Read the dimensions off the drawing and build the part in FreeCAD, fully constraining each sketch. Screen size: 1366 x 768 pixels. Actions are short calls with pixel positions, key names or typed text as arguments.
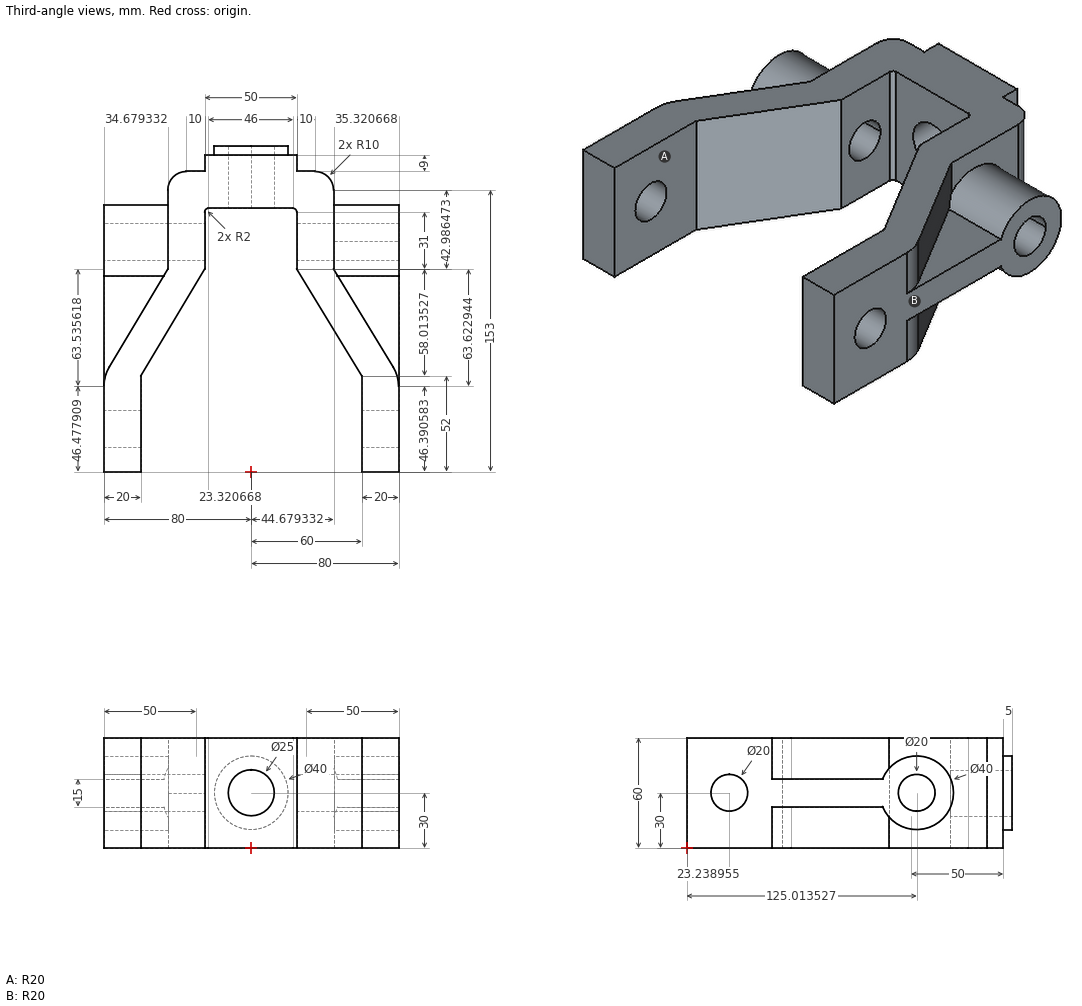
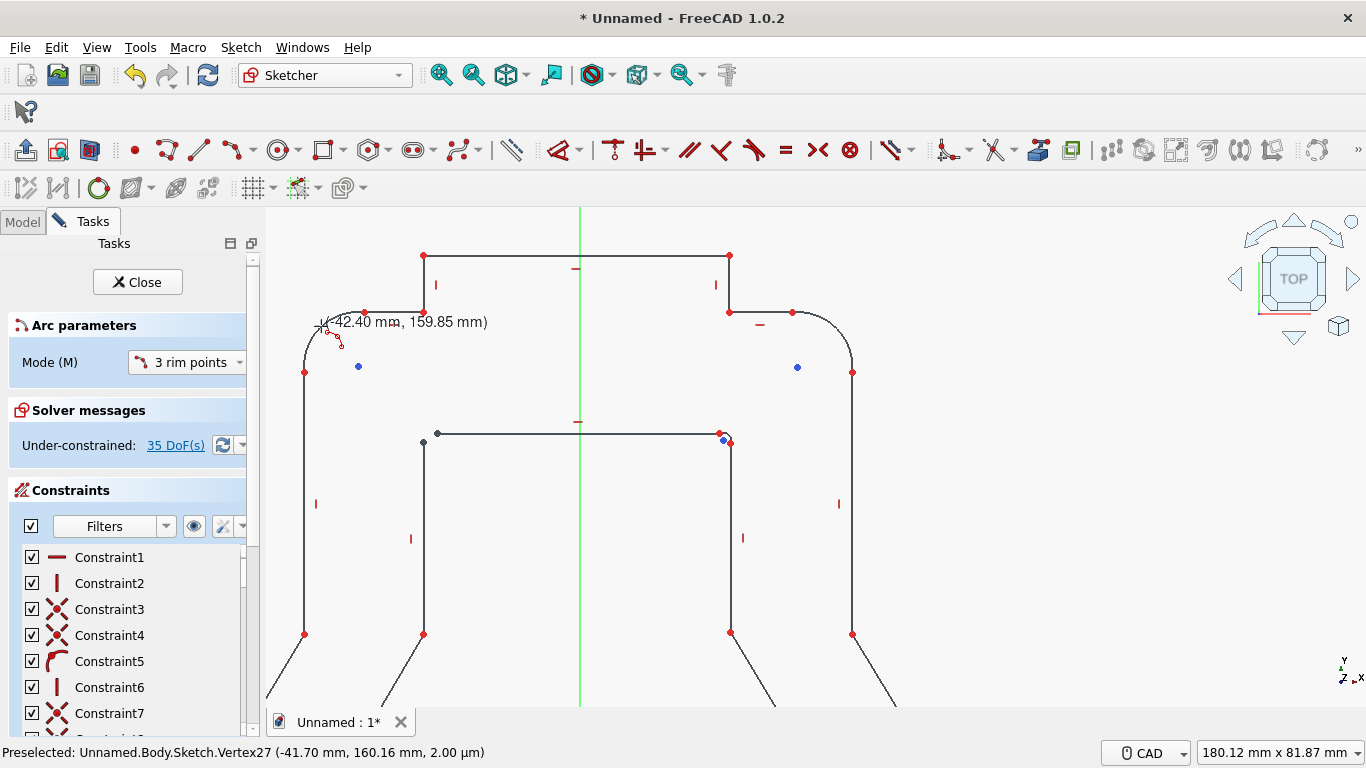
click(424, 443)
click(437, 434)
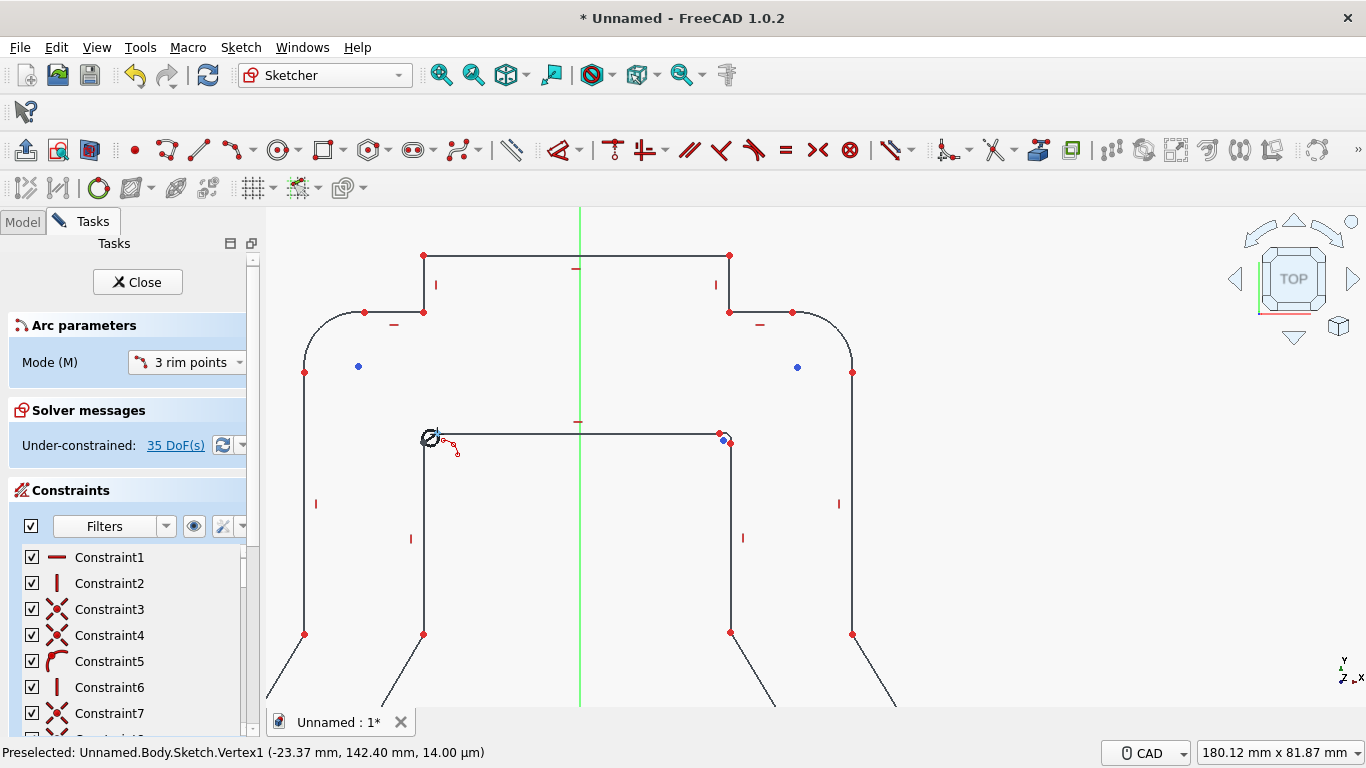
scroll(429, 433, up, 8)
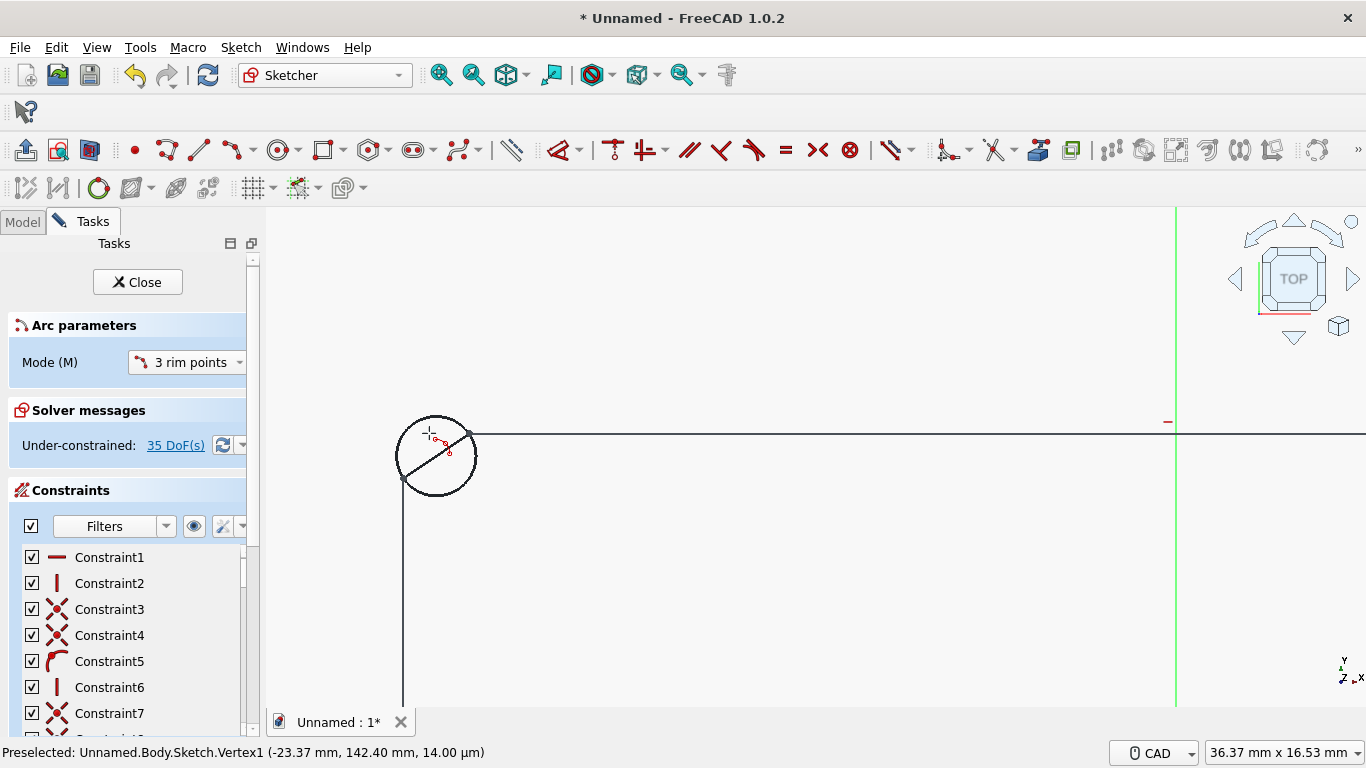
click(428, 433)
key(Escape)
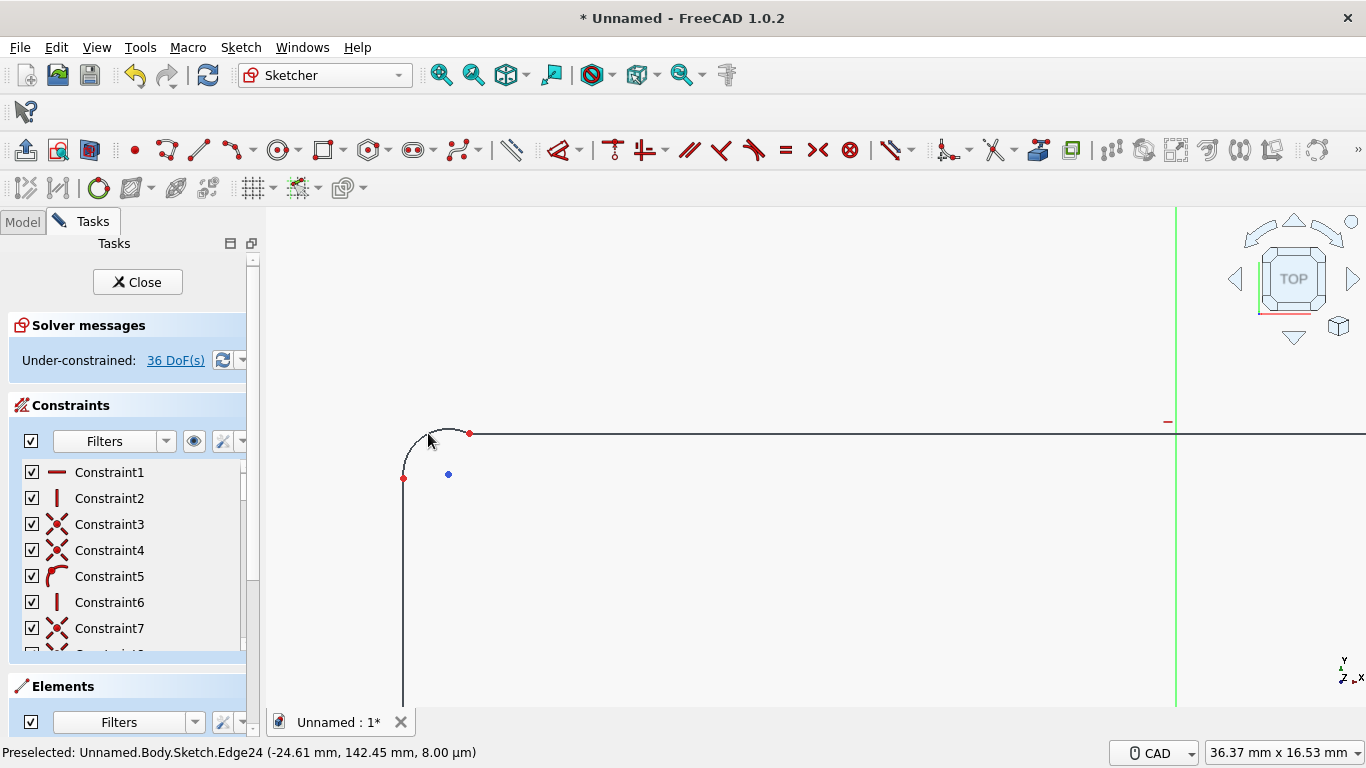
scroll(720, 348, down, 14)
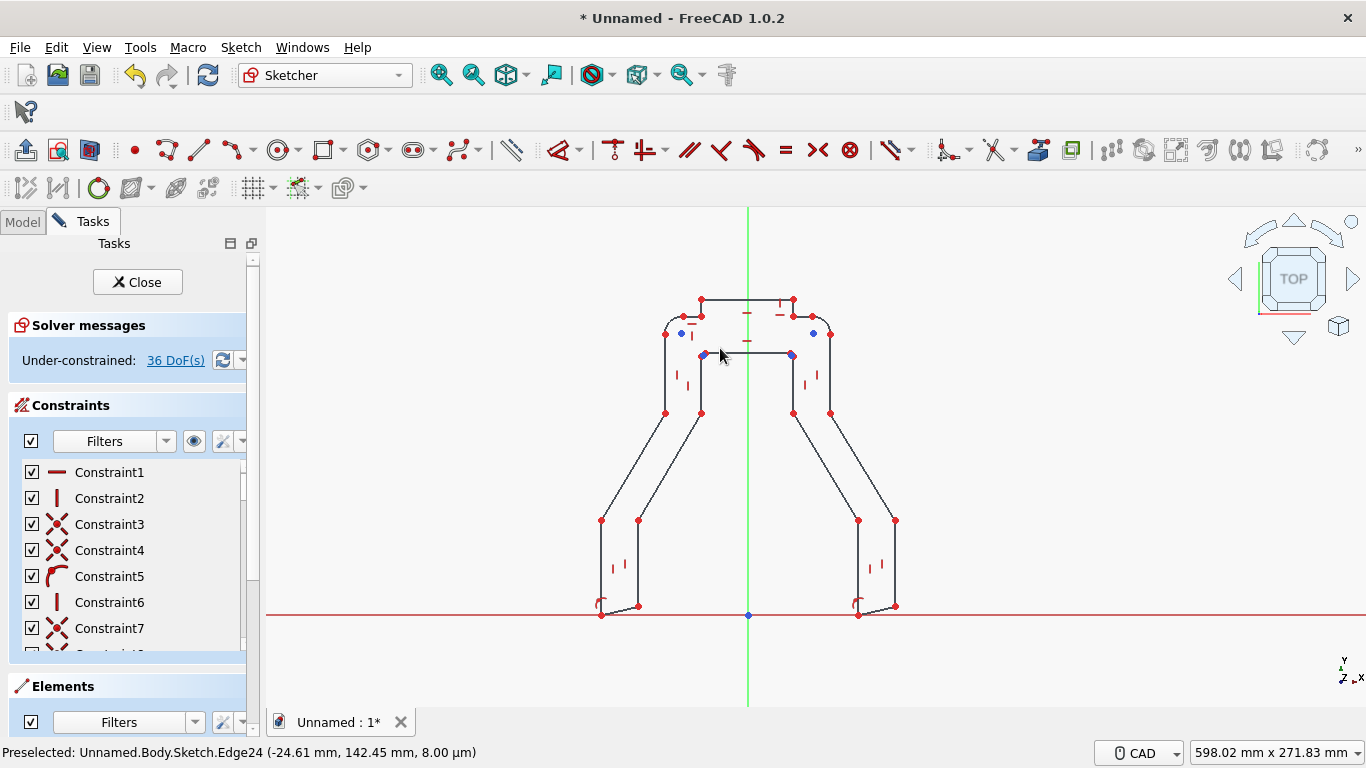
click(731, 353)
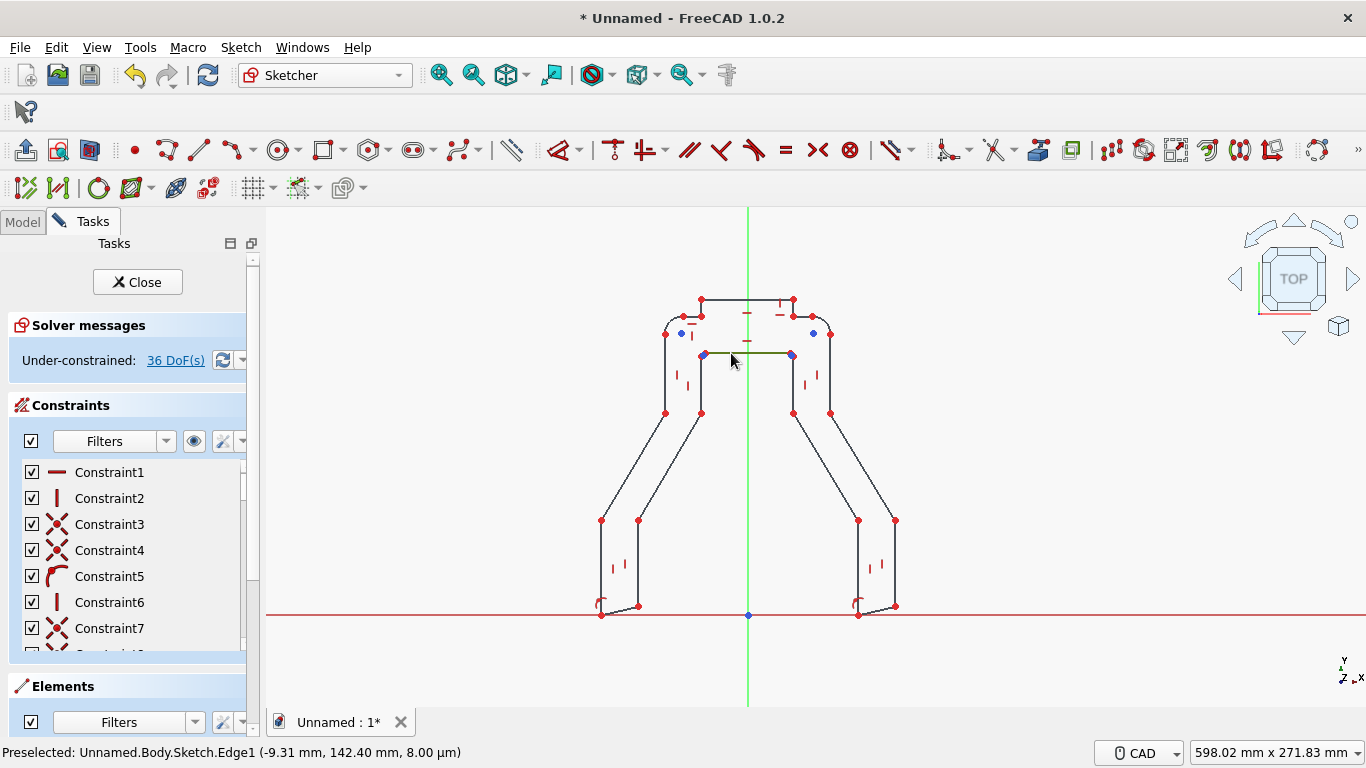
scroll(793, 354, up, 9)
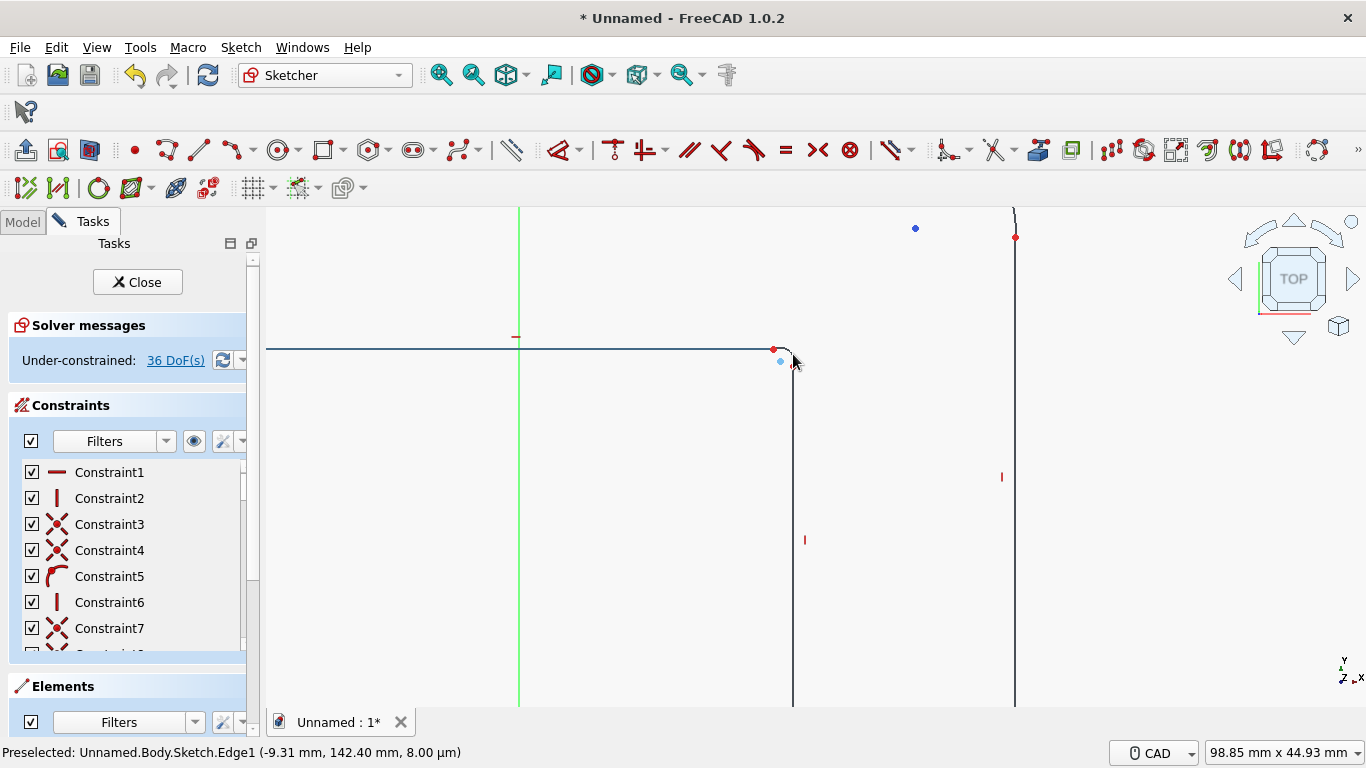
click(789, 351)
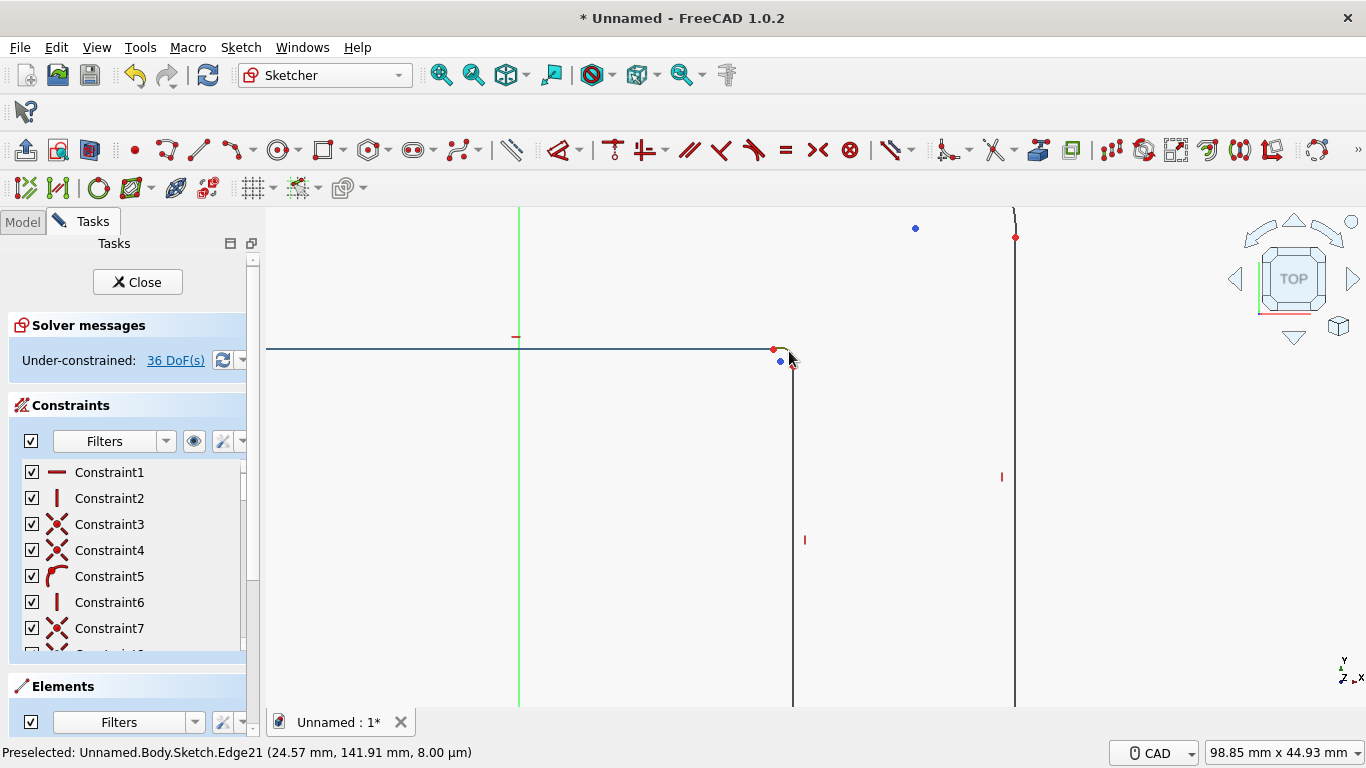
key(t)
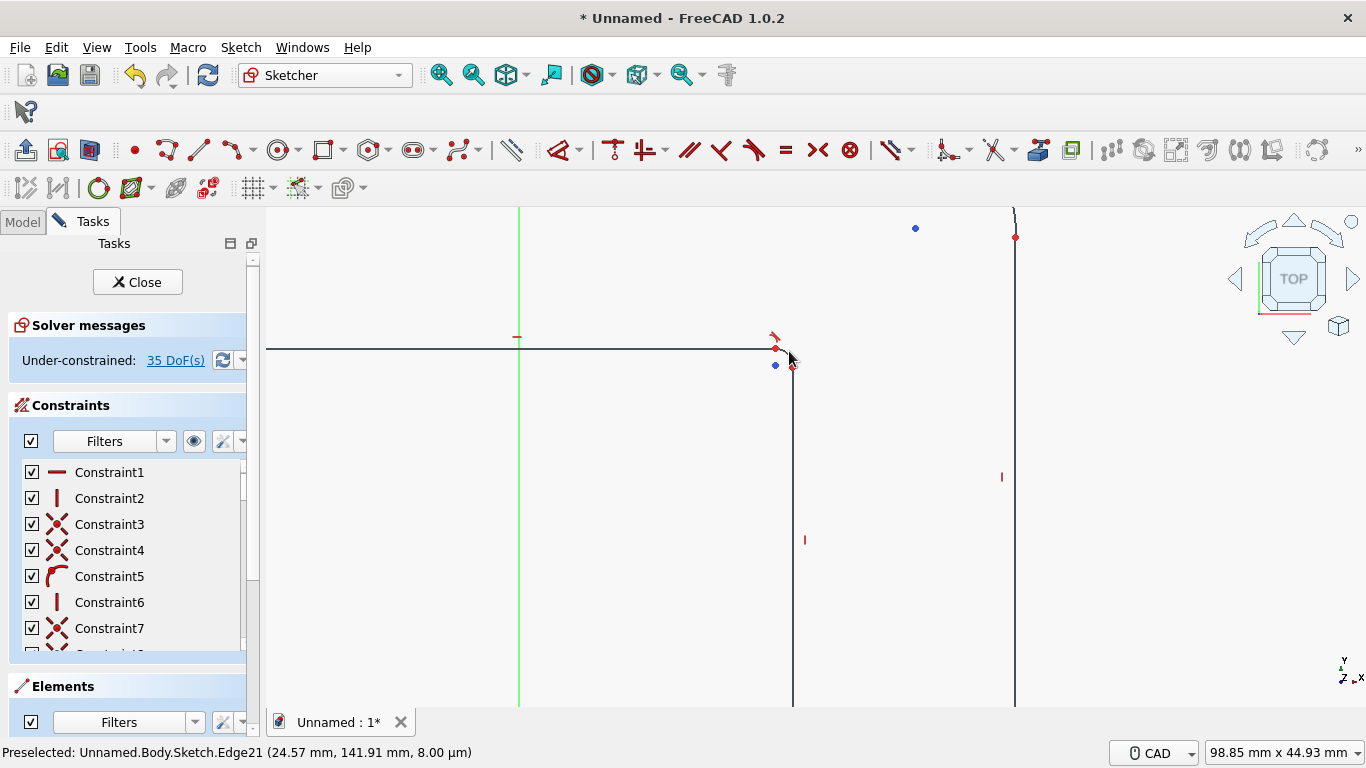
scroll(793, 354, down, 9)